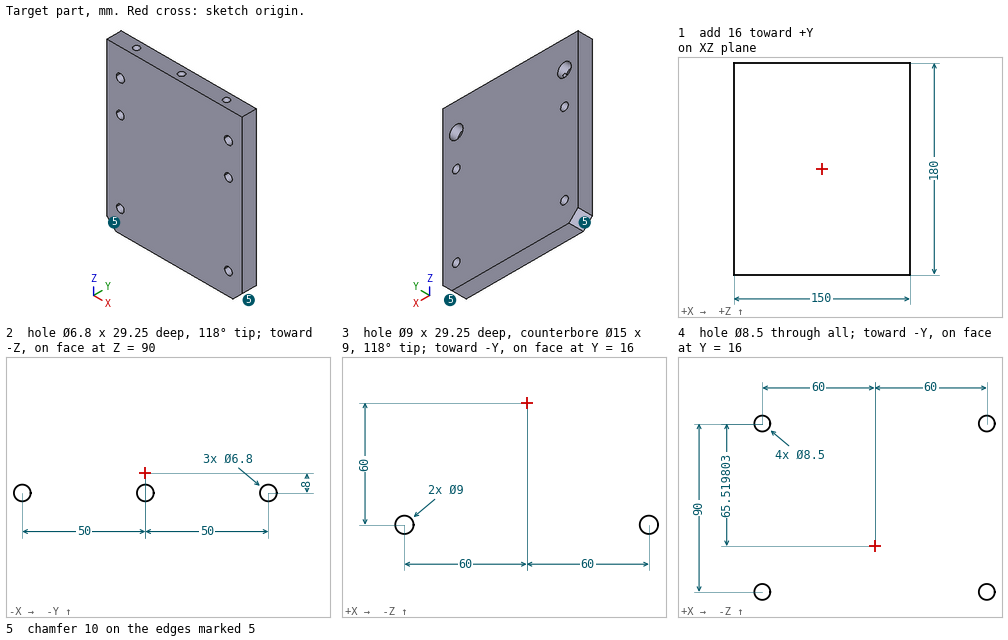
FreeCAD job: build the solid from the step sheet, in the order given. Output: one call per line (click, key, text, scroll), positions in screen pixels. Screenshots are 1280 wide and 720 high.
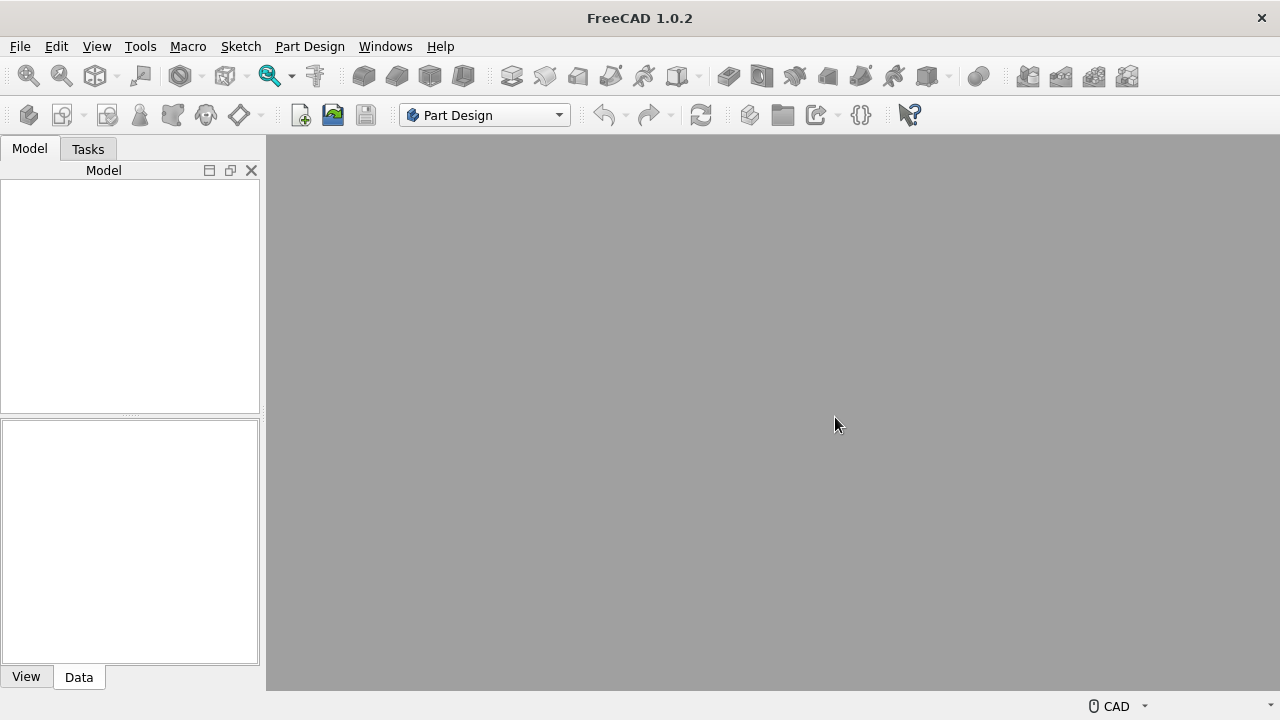
click(300, 116)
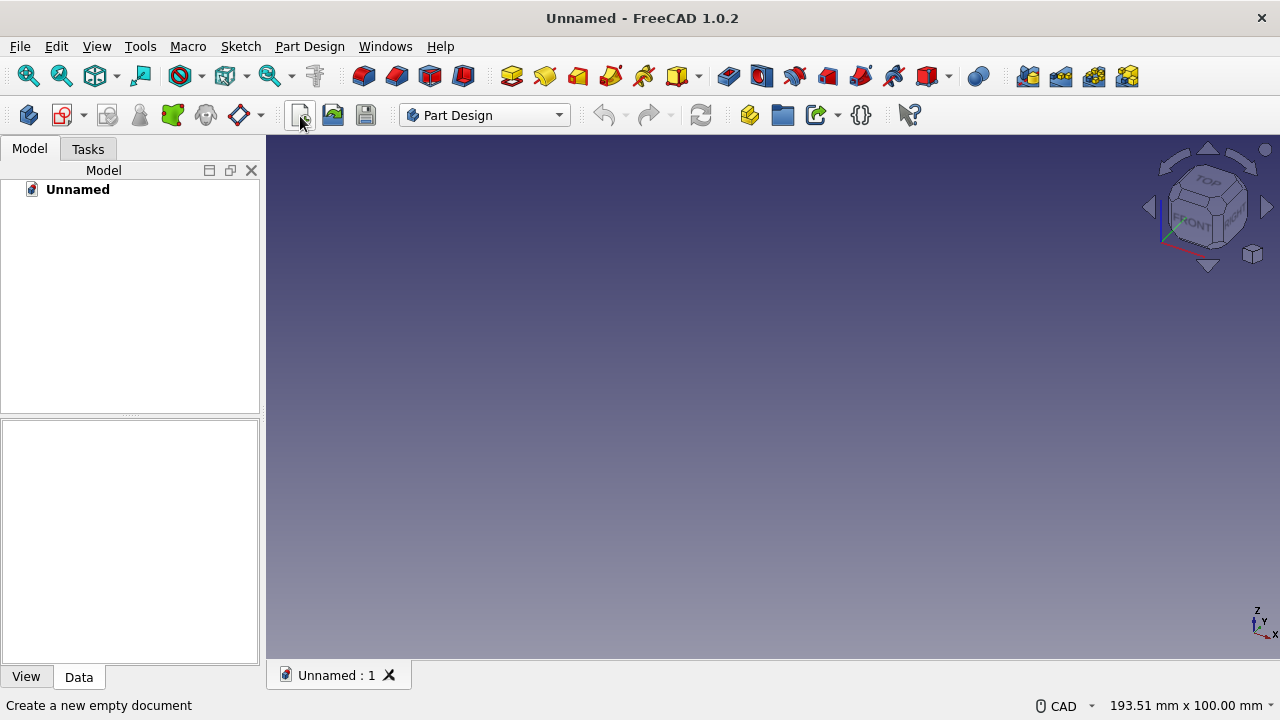
click(62, 116)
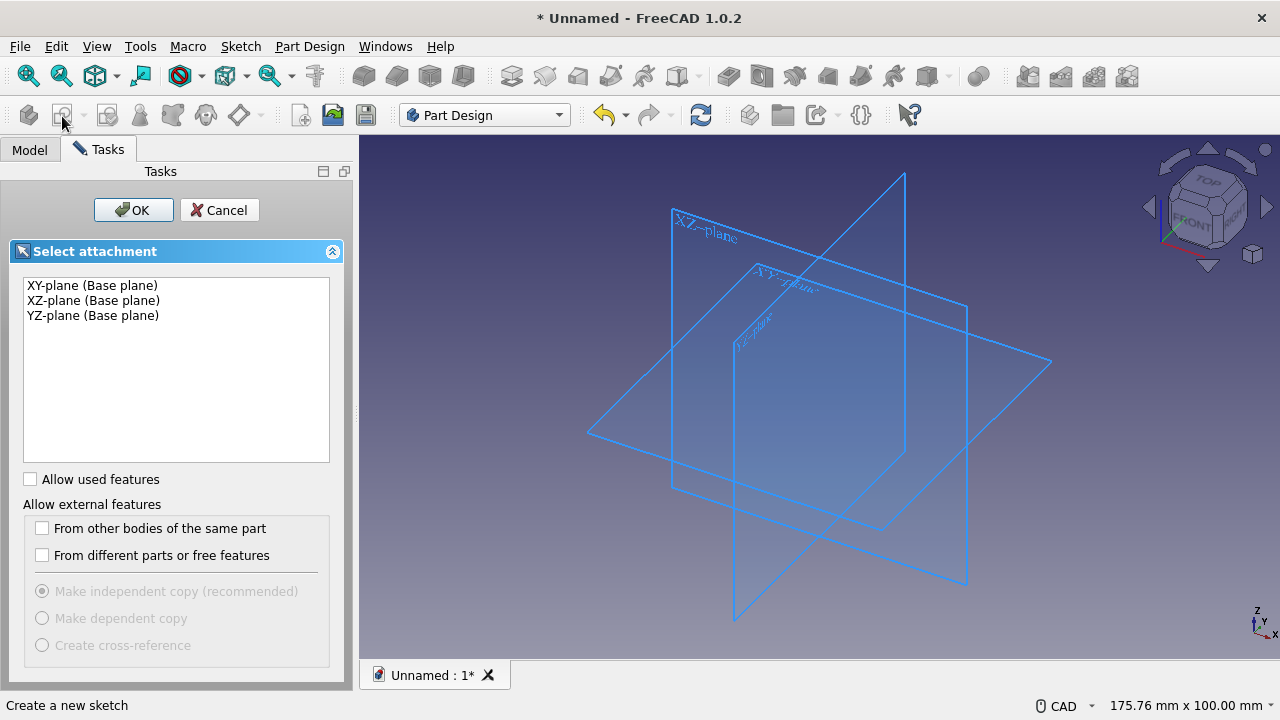
click(84, 300)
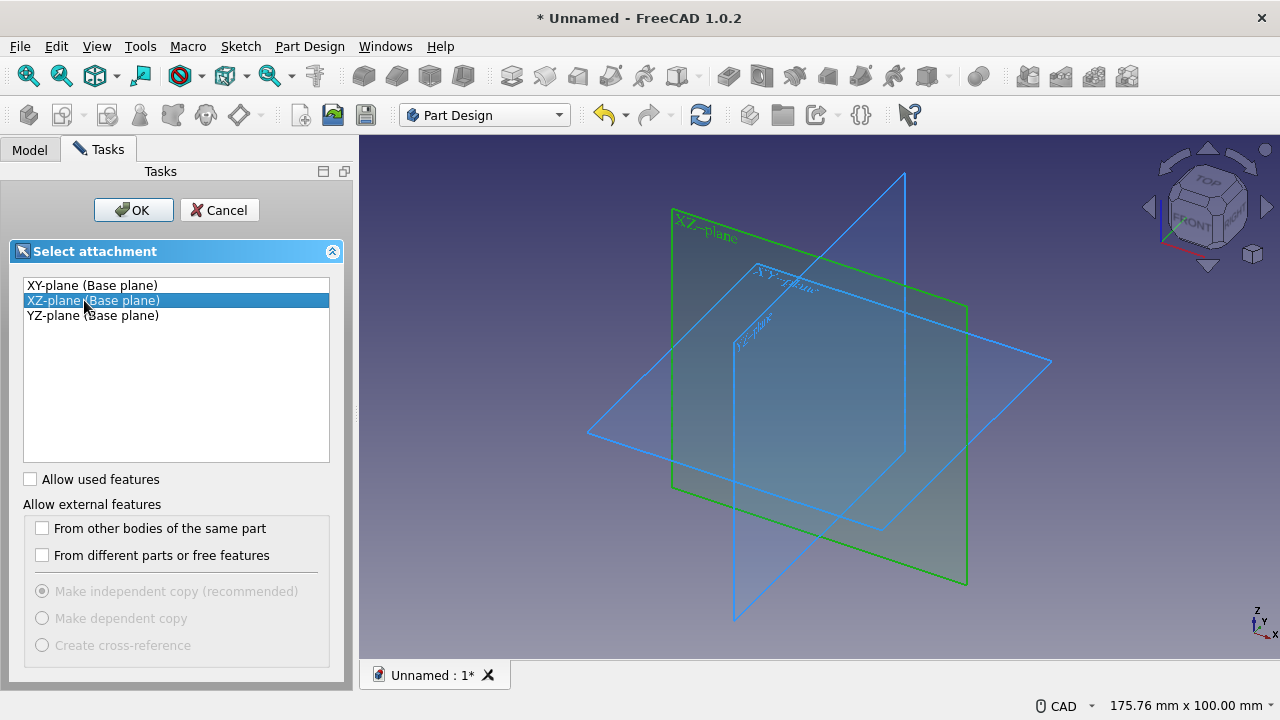
click(134, 210)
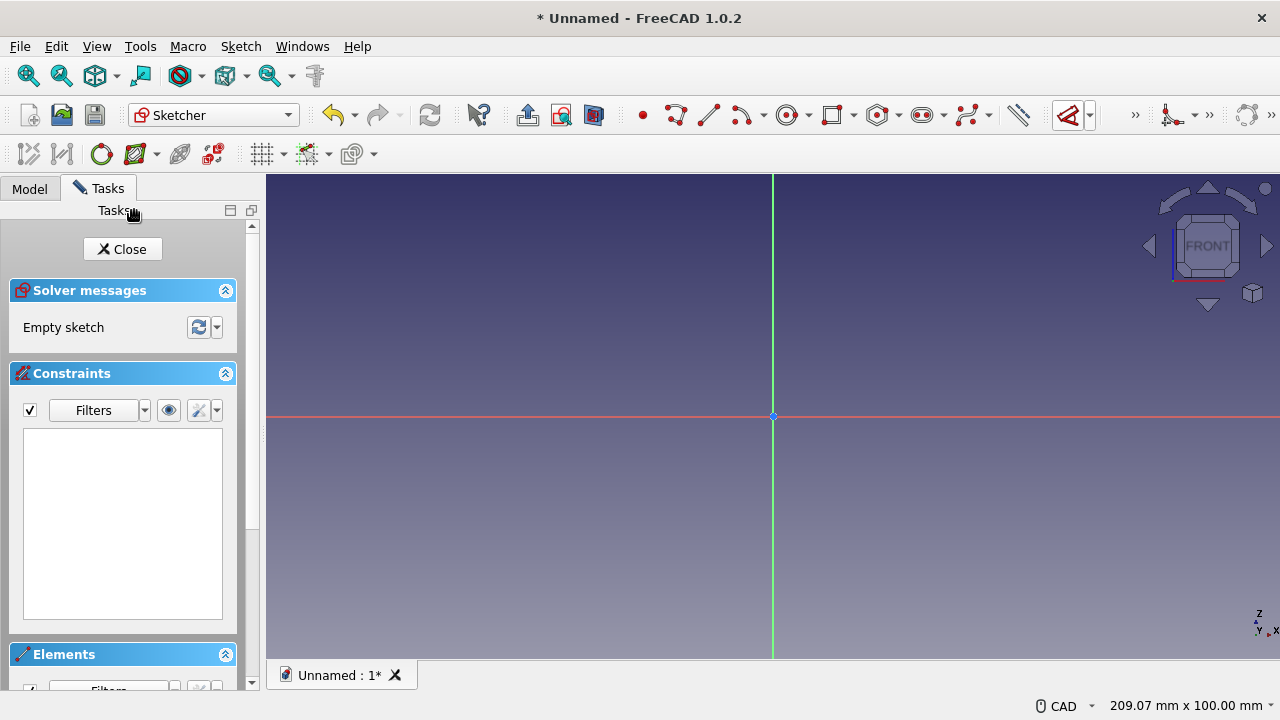
scroll(665, 417, down, 5)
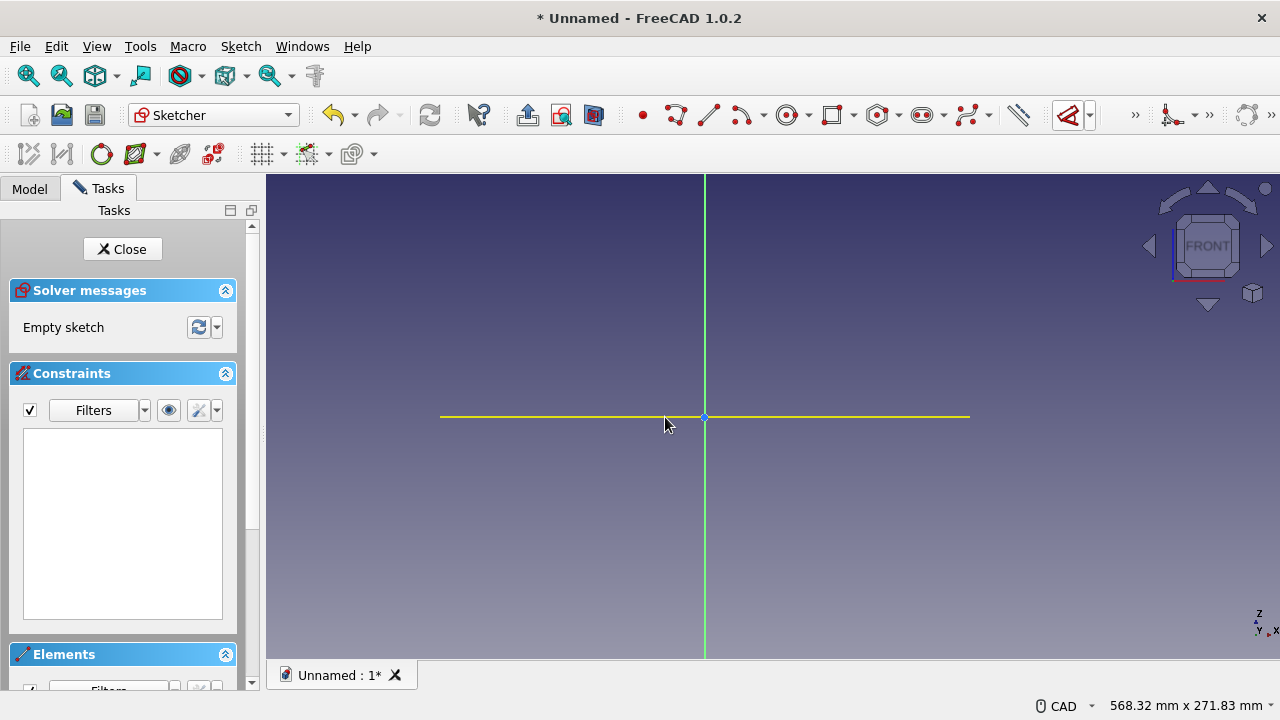
click(854, 116)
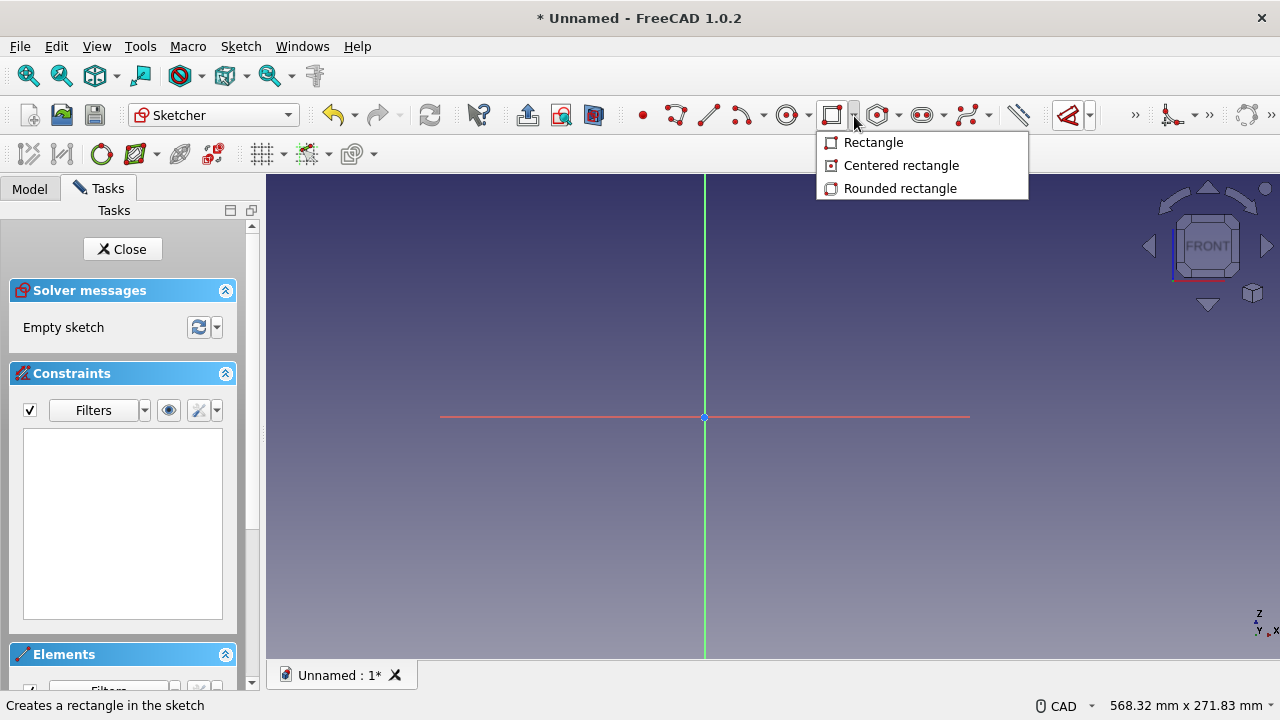
click(922, 166)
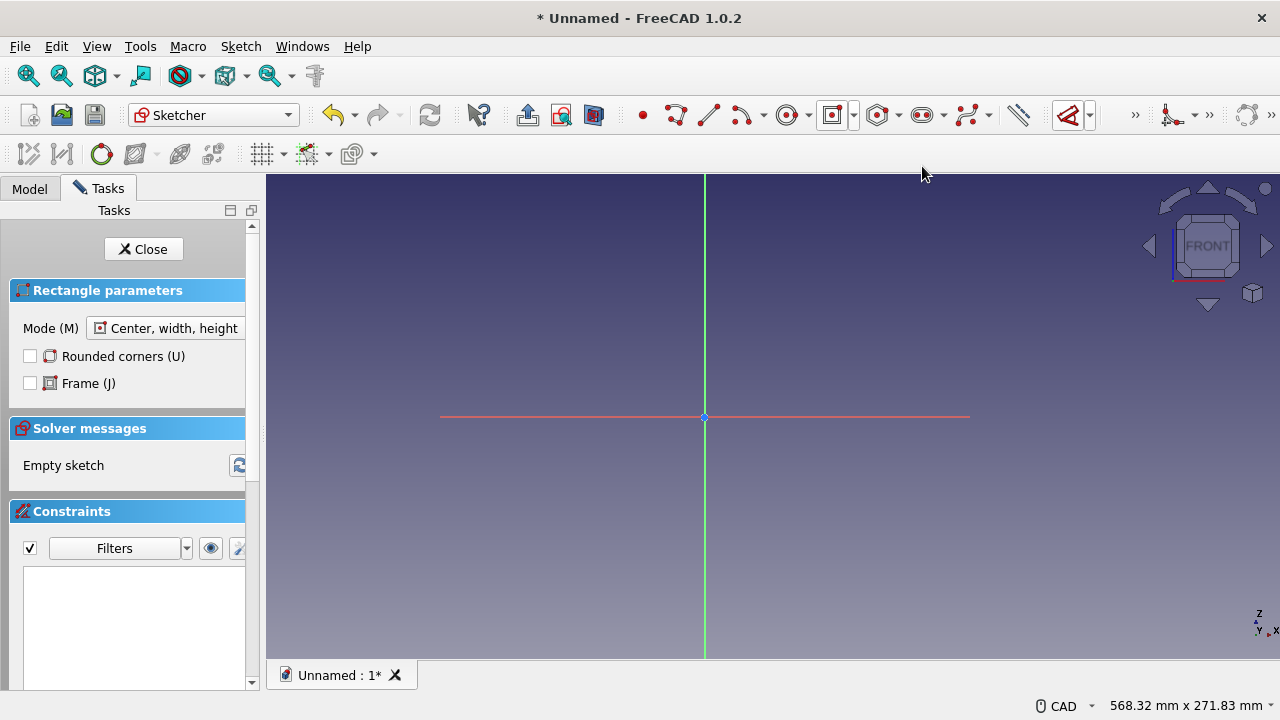
click(705, 417)
move(839, 257)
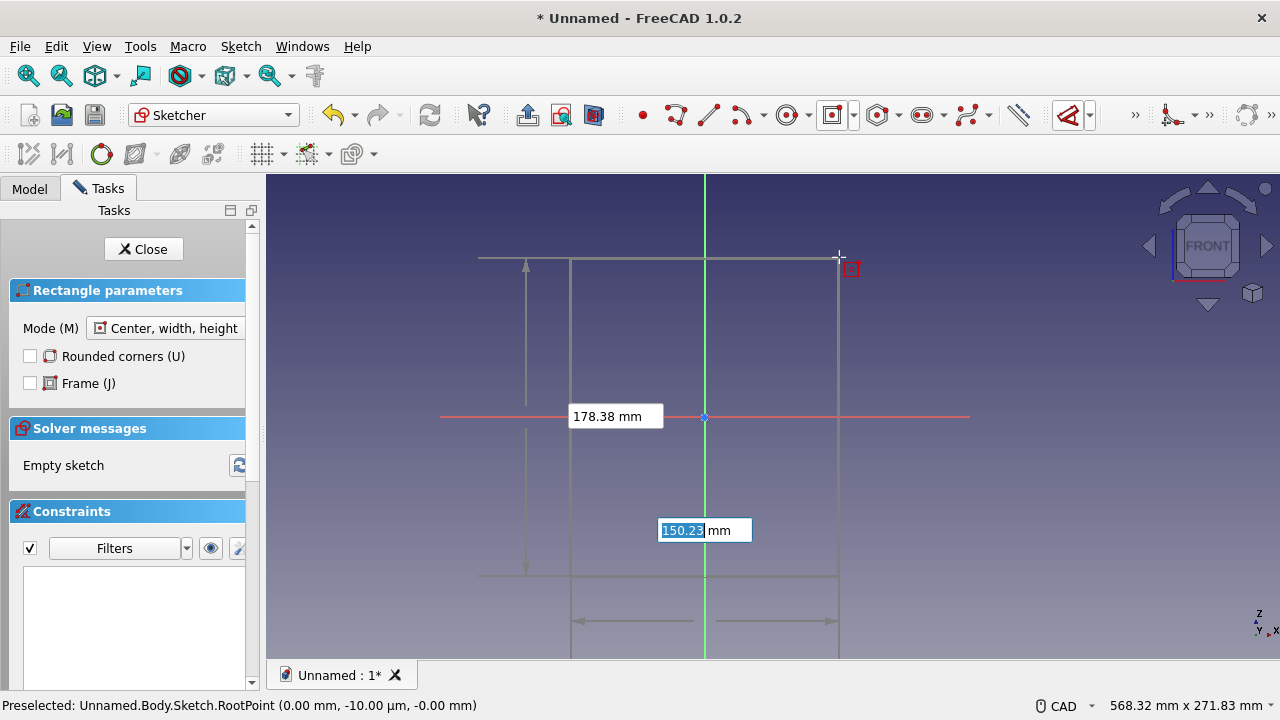
text(150)
key(Tab)
text(180)
key(Return)
key(Escape)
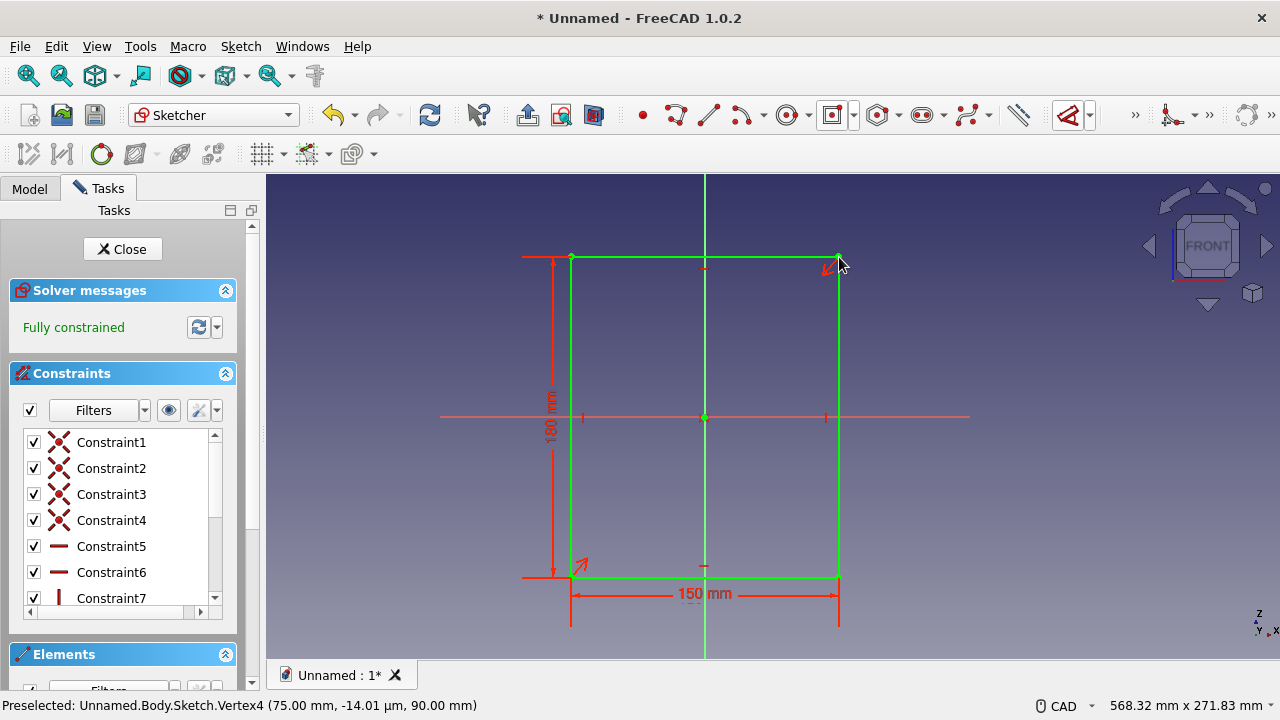
click(123, 249)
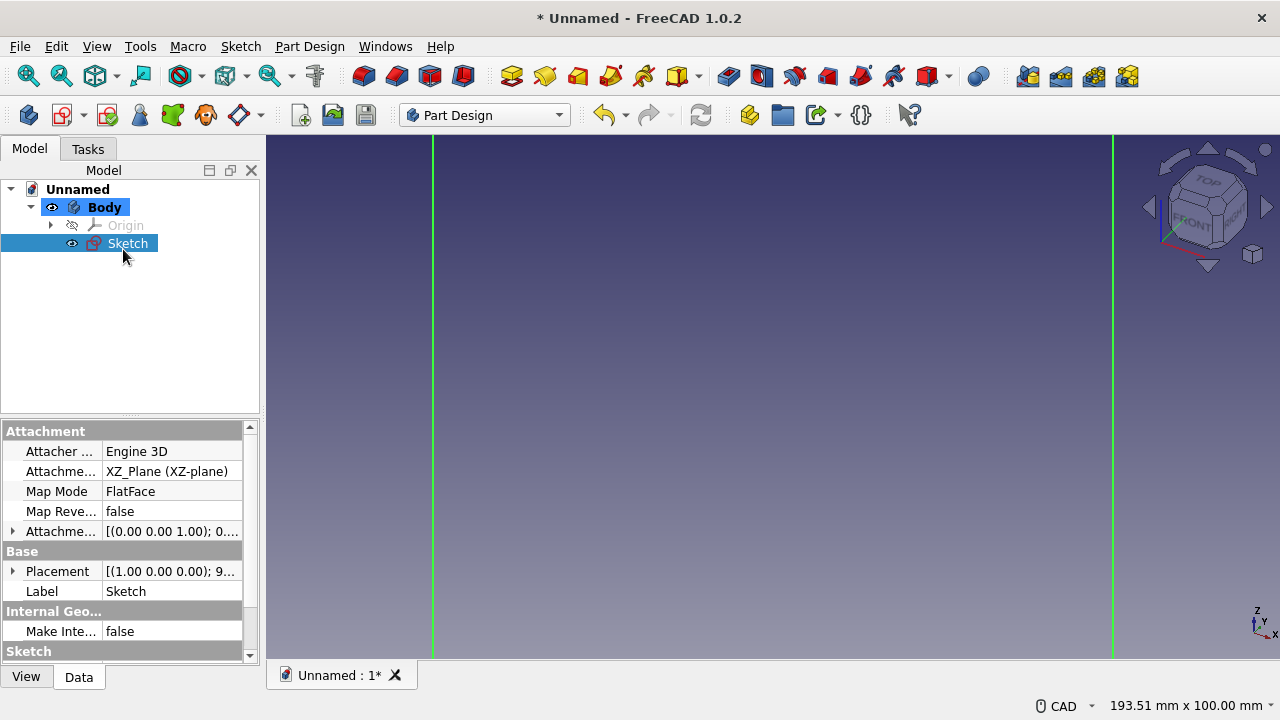
click(512, 76)